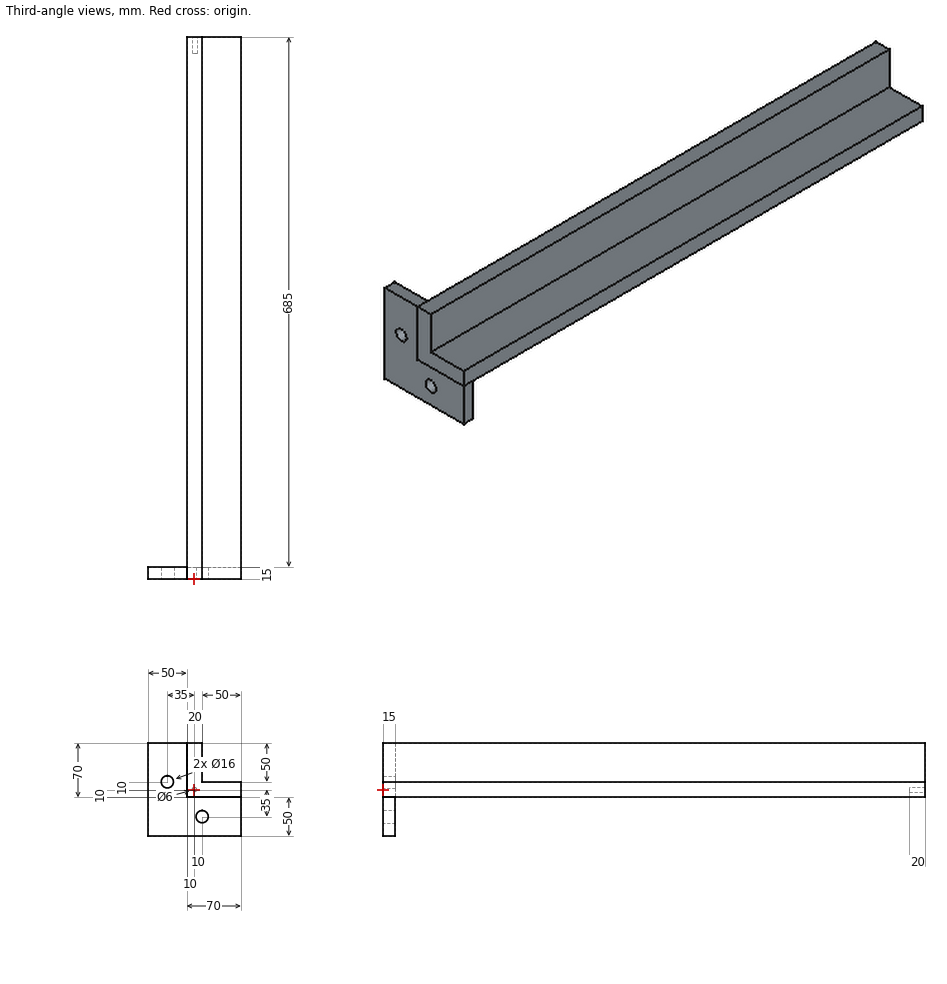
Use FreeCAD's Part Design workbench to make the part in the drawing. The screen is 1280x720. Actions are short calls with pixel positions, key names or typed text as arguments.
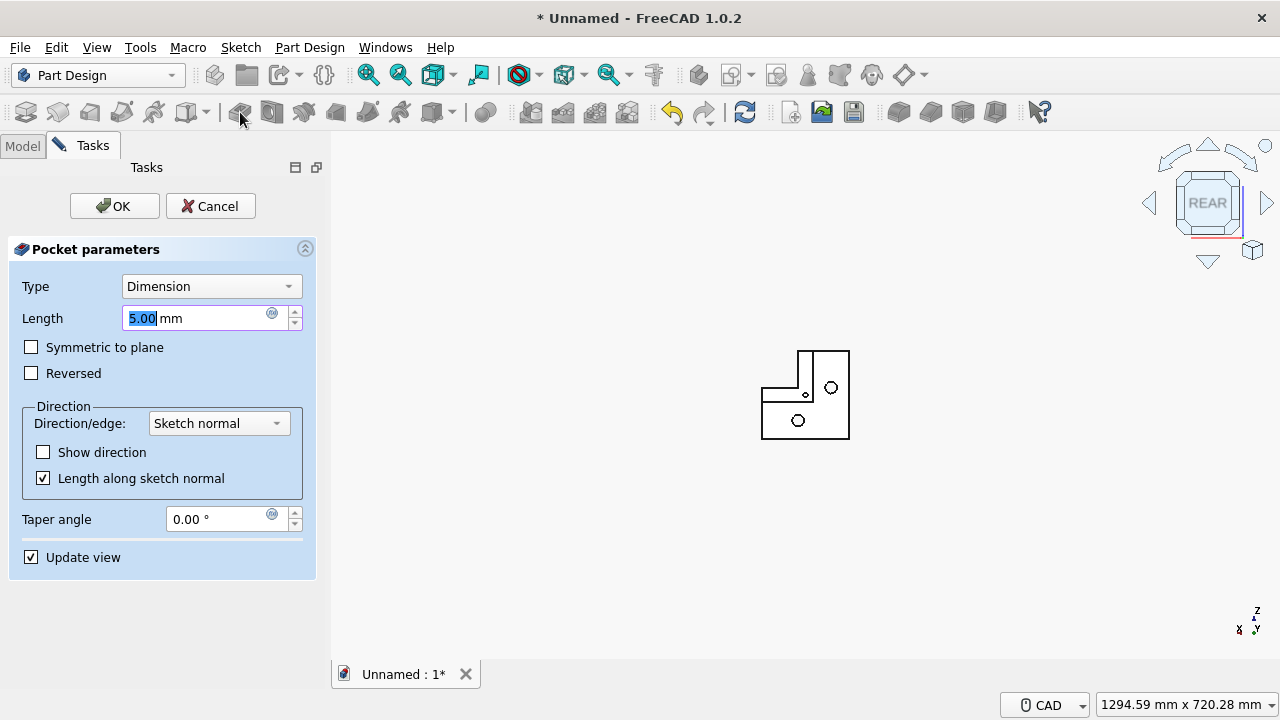
text(20)
key(Tab)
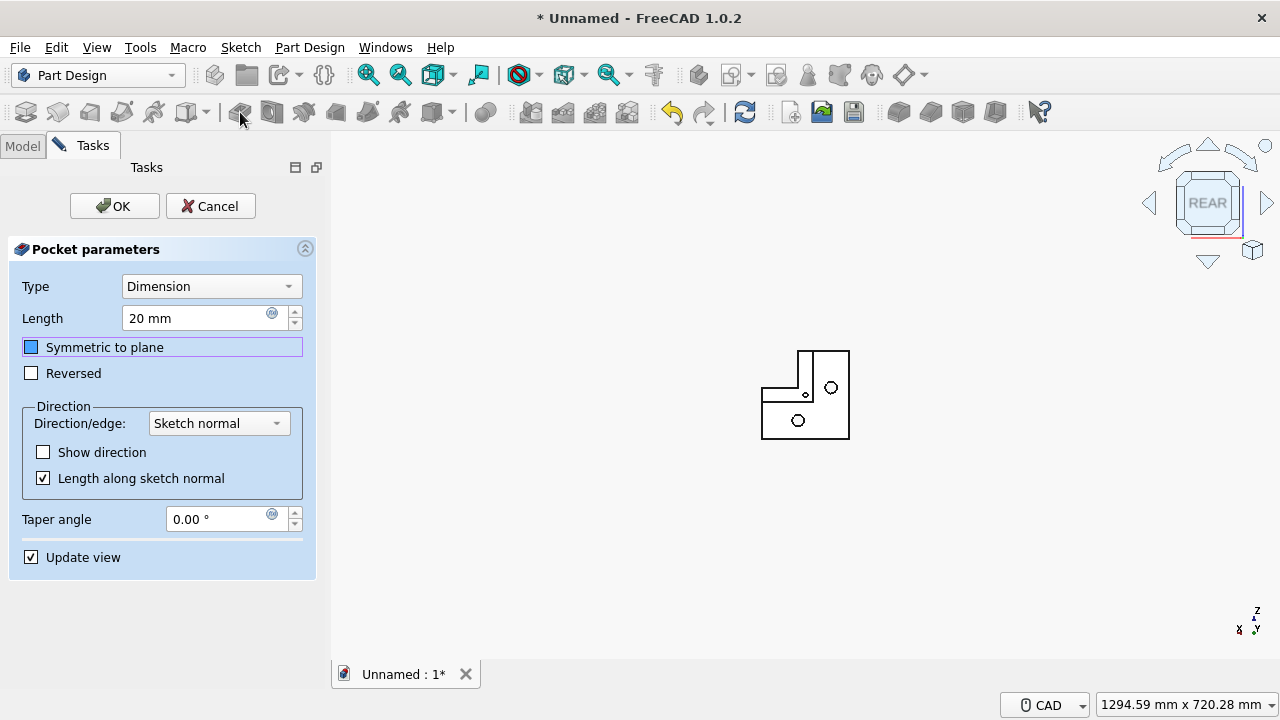
click(115, 206)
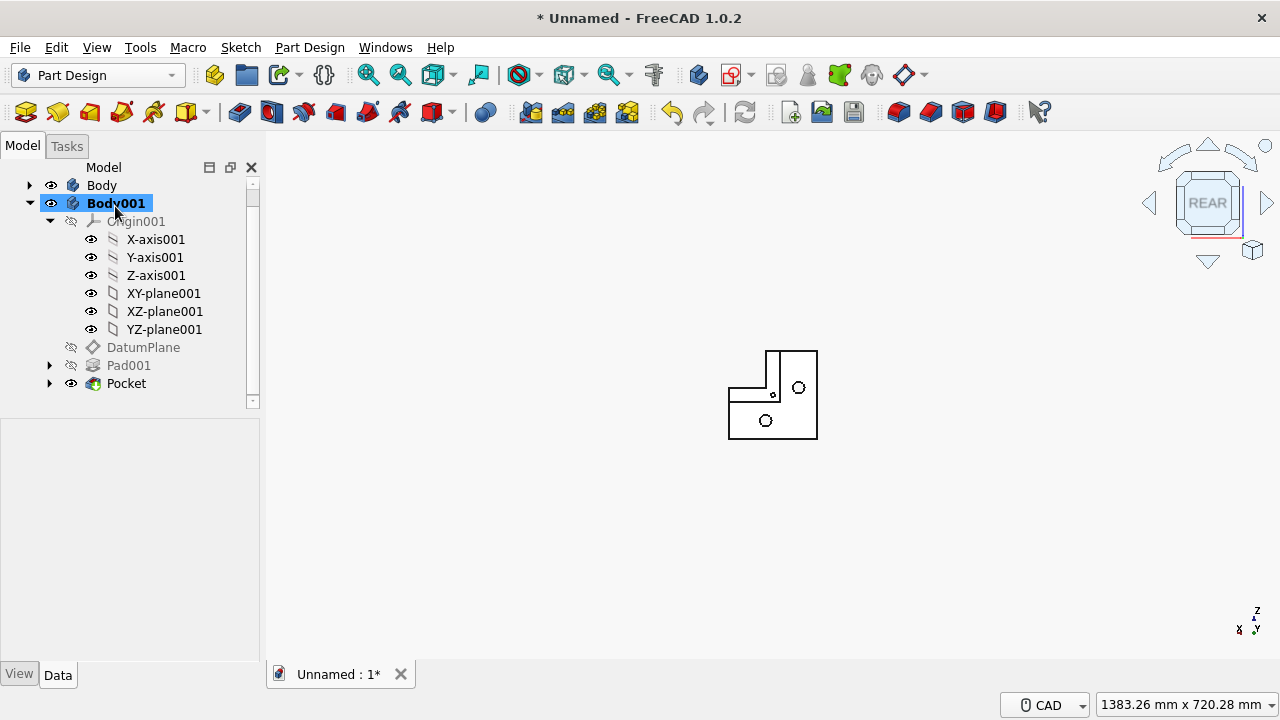
key(0)